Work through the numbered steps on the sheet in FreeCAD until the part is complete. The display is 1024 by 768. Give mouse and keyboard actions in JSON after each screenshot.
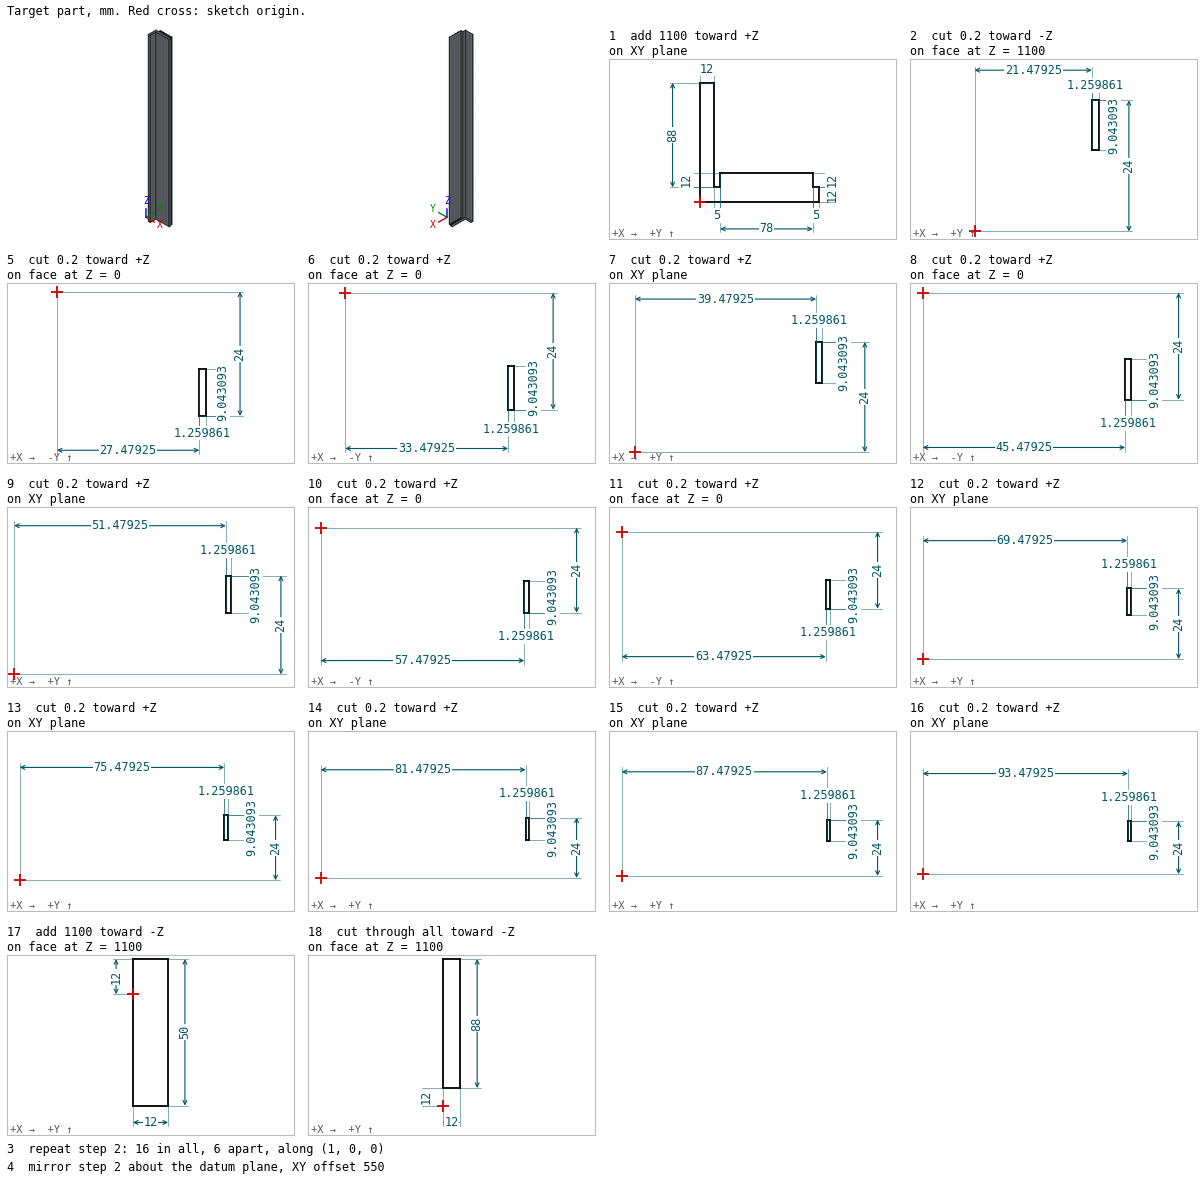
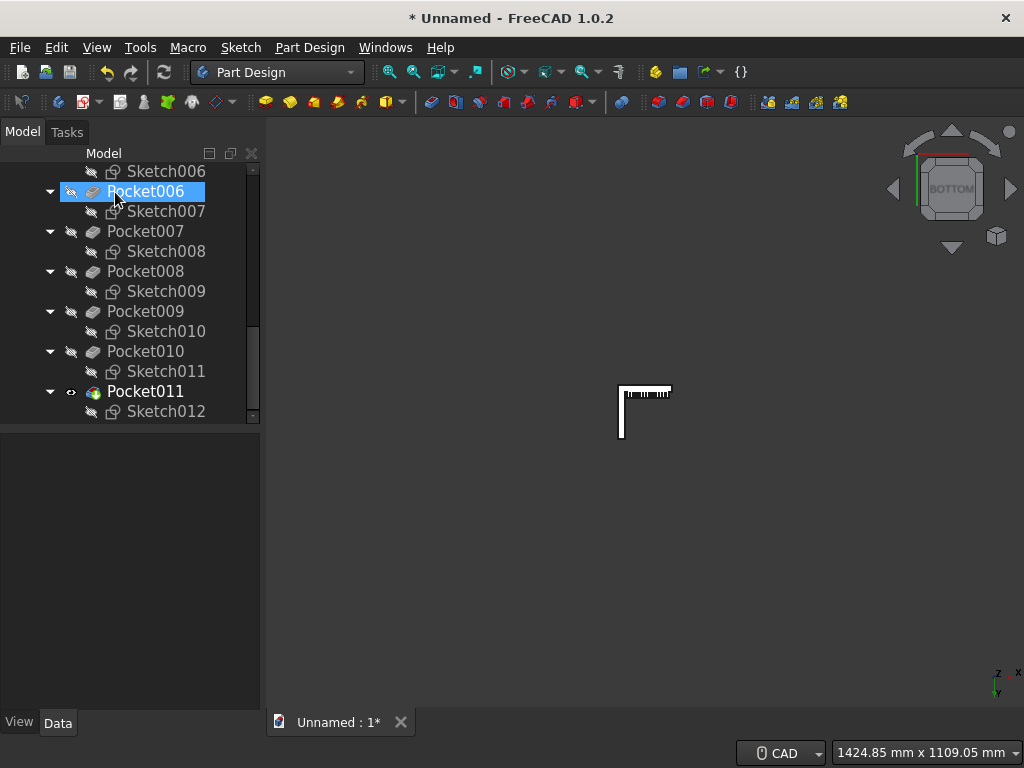
{"action": "left_click", "coordinate": [390, 72]}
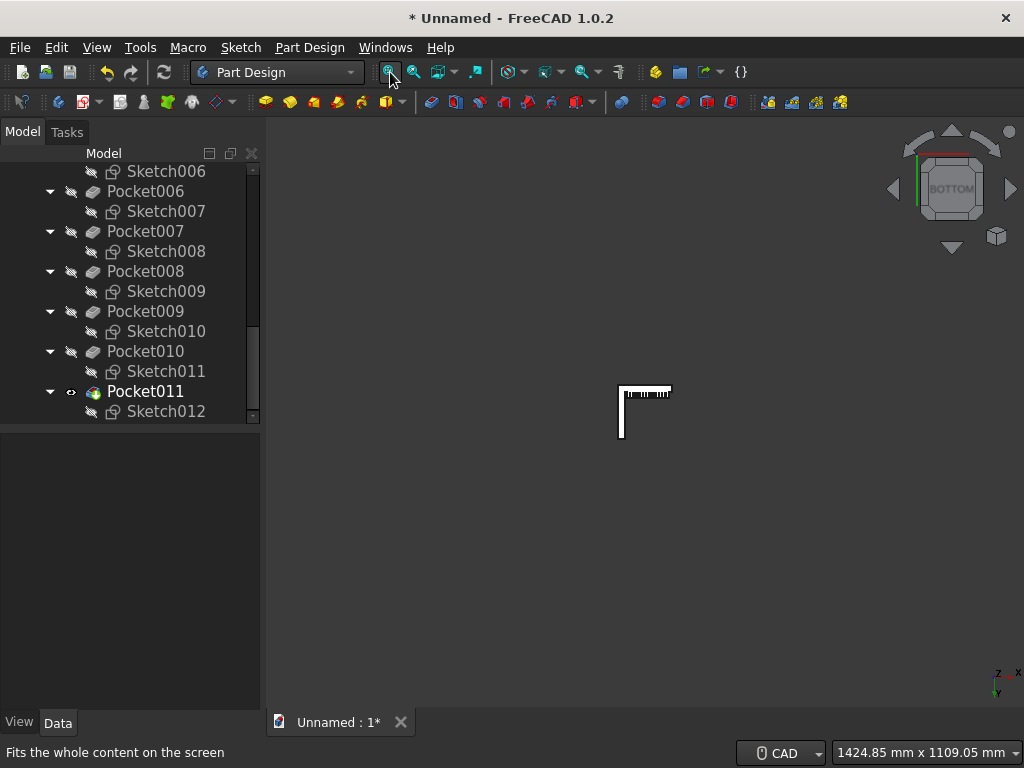
{"action": "left_click", "coordinate": [84, 102]}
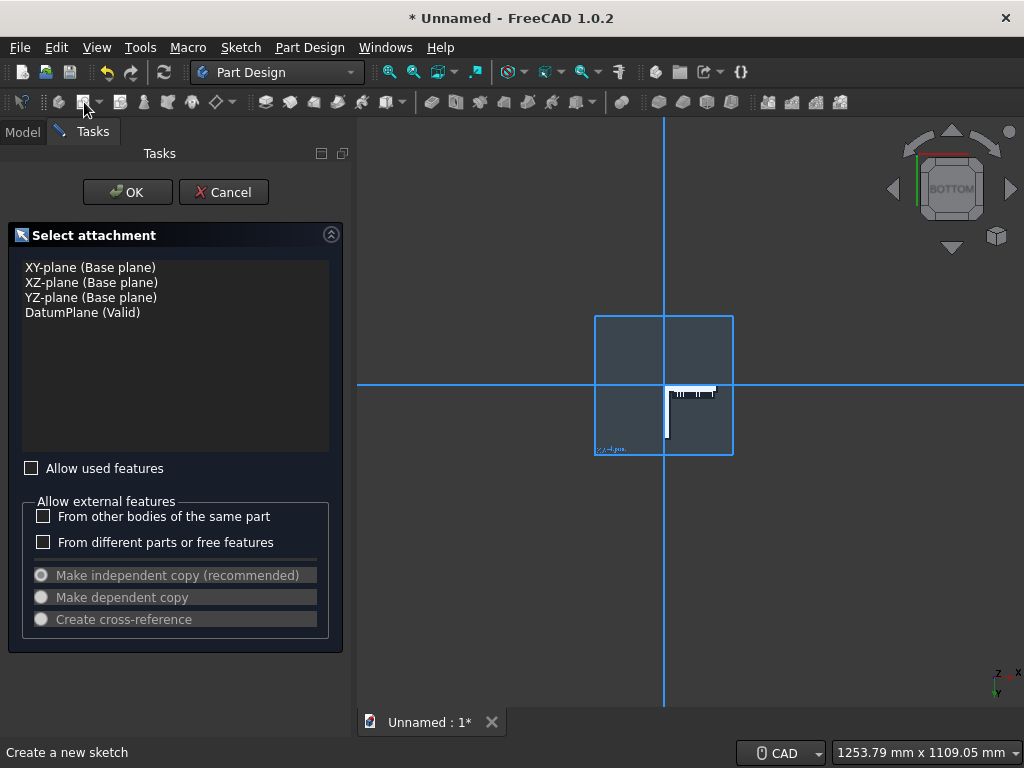
{"action": "left_click", "coordinate": [82, 268]}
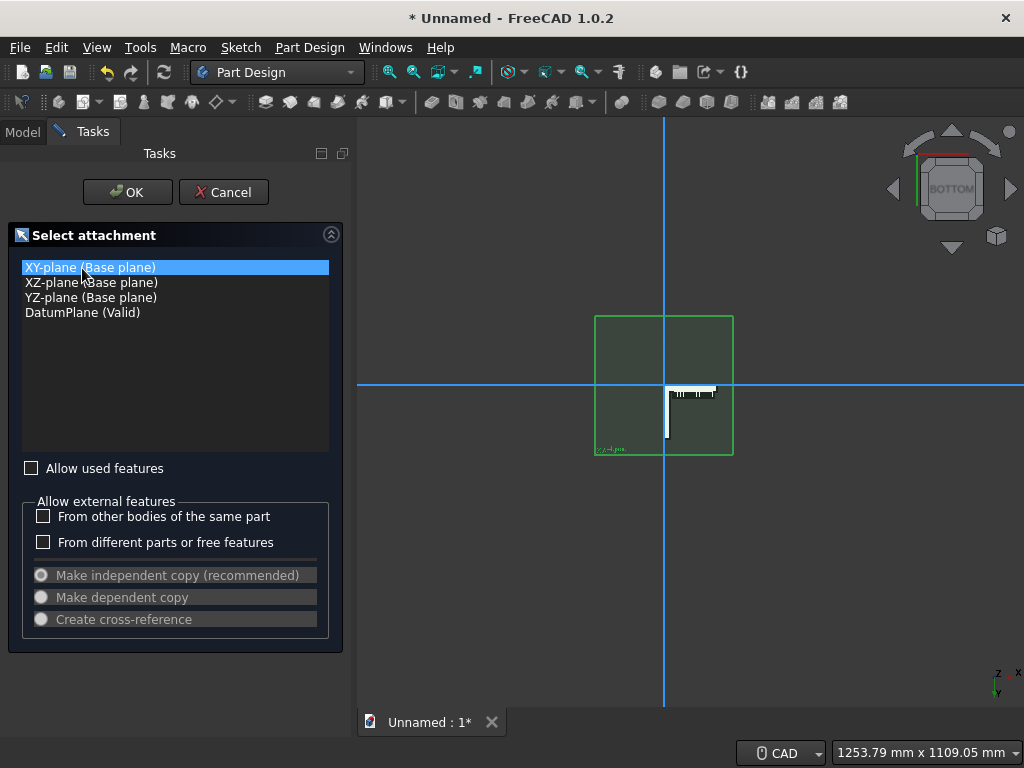
{"action": "left_click", "coordinate": [128, 192]}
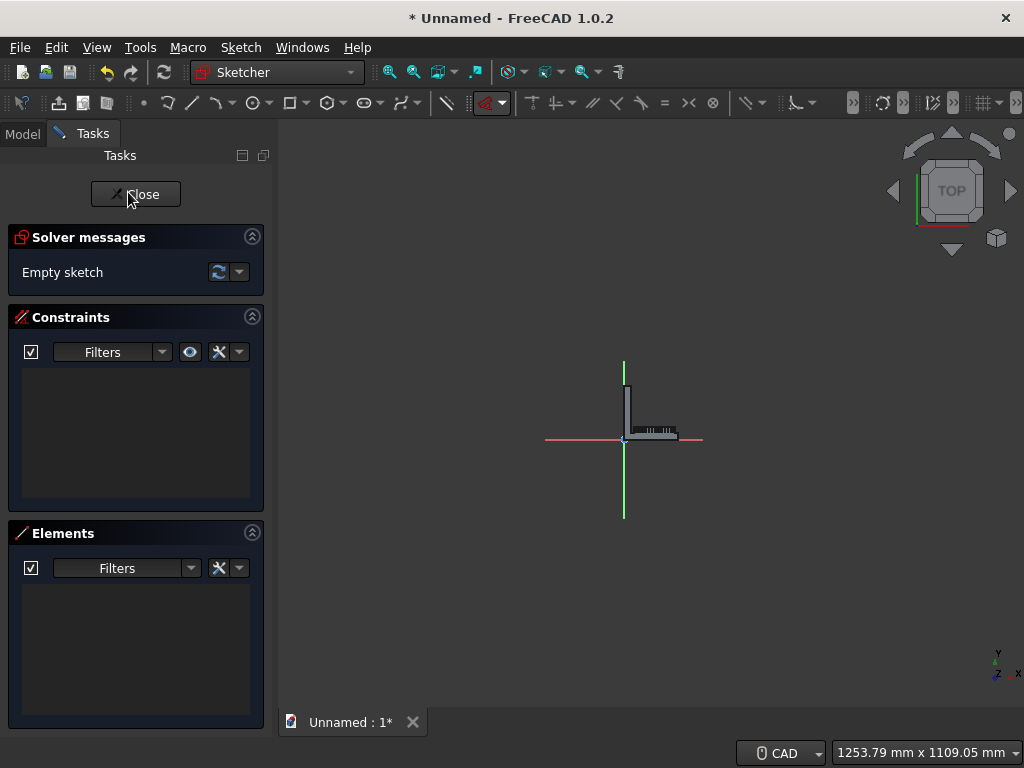
{"action": "left_click", "coordinate": [108, 104]}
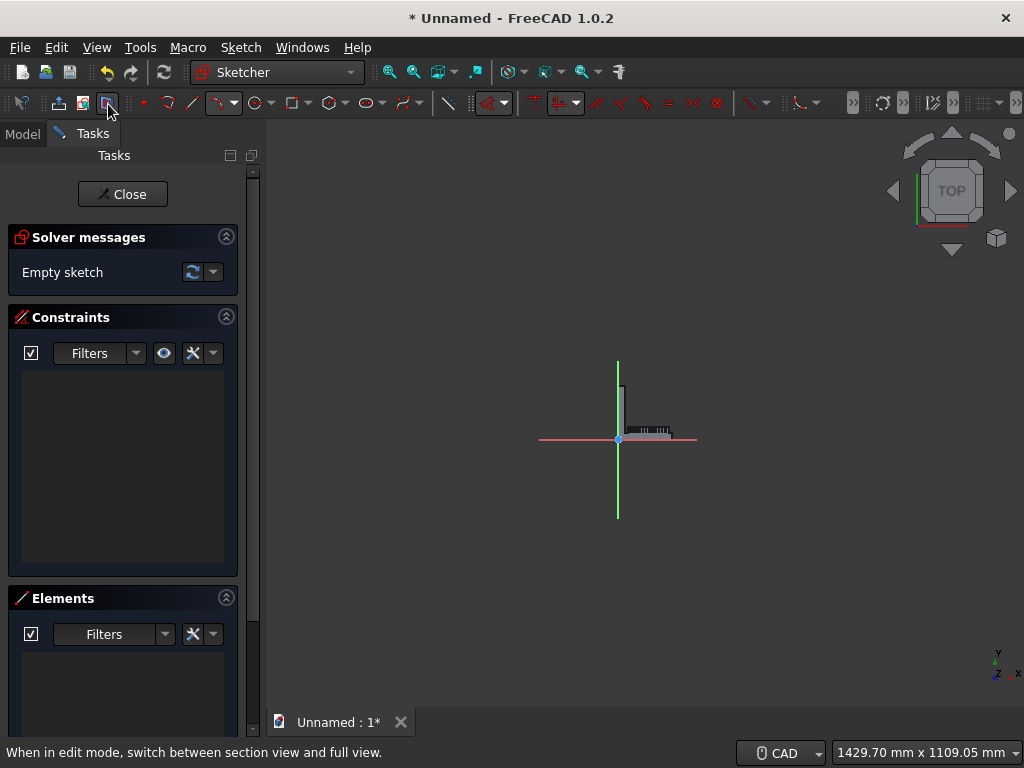
{"action": "scroll", "coordinate": [673, 430], "scroll_direction": "up", "scroll_amount": 15}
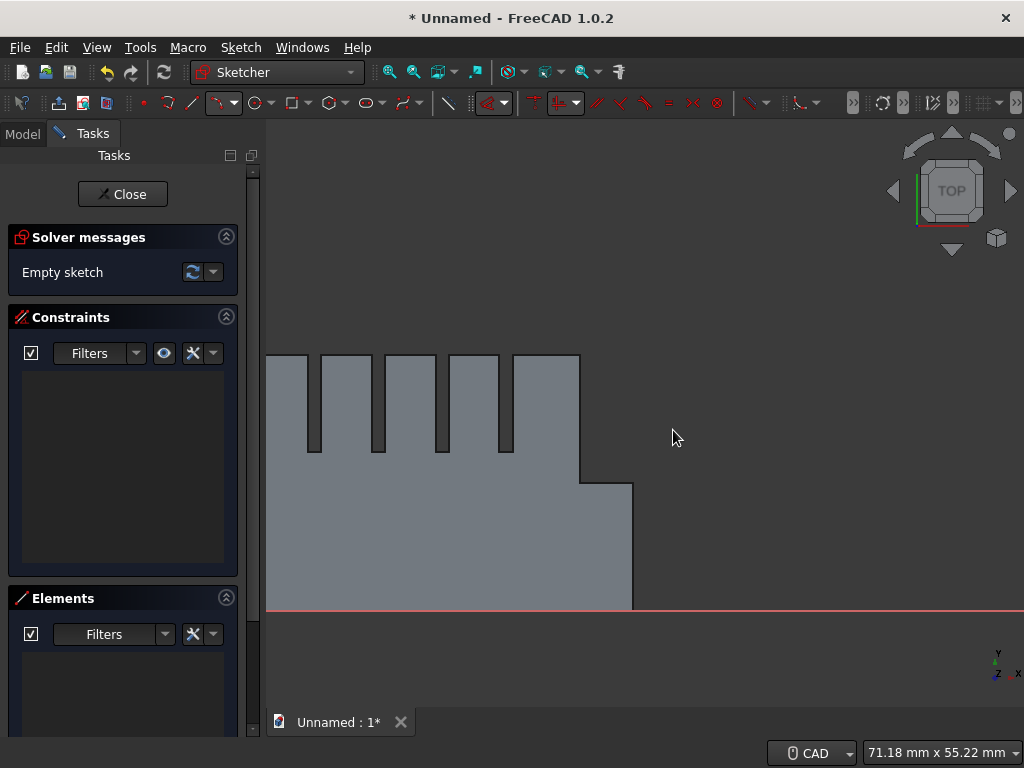
{"action": "scroll", "coordinate": [568, 400], "scroll_direction": "up", "scroll_amount": 7}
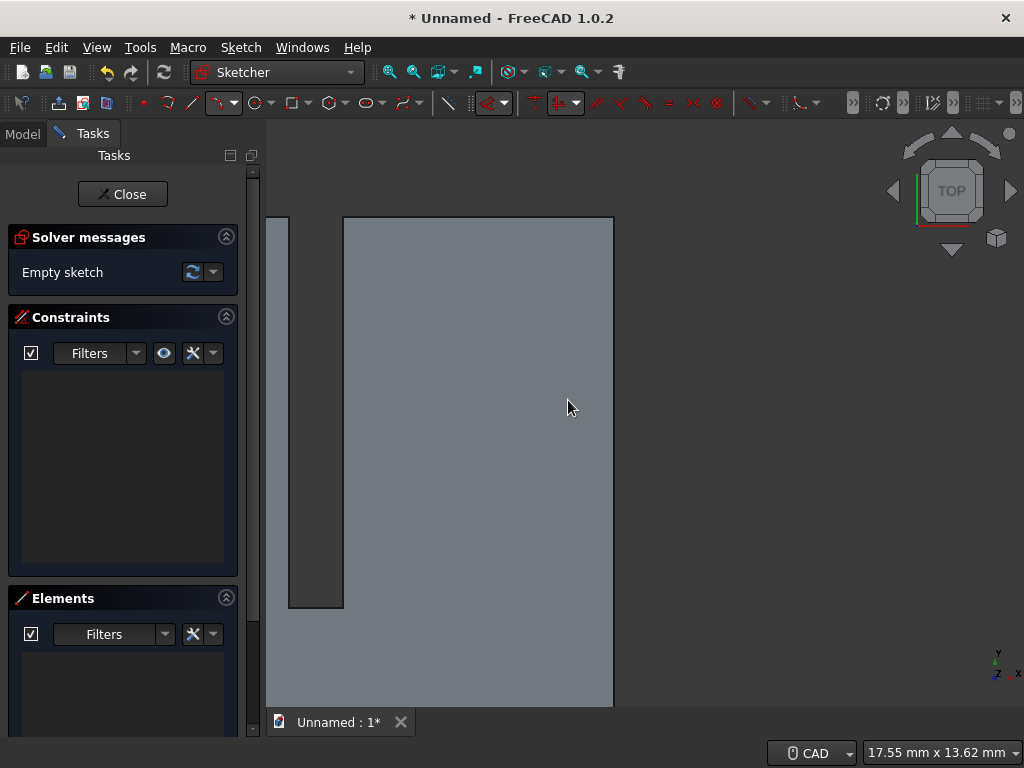
{"action": "left_click", "coordinate": [292, 104]}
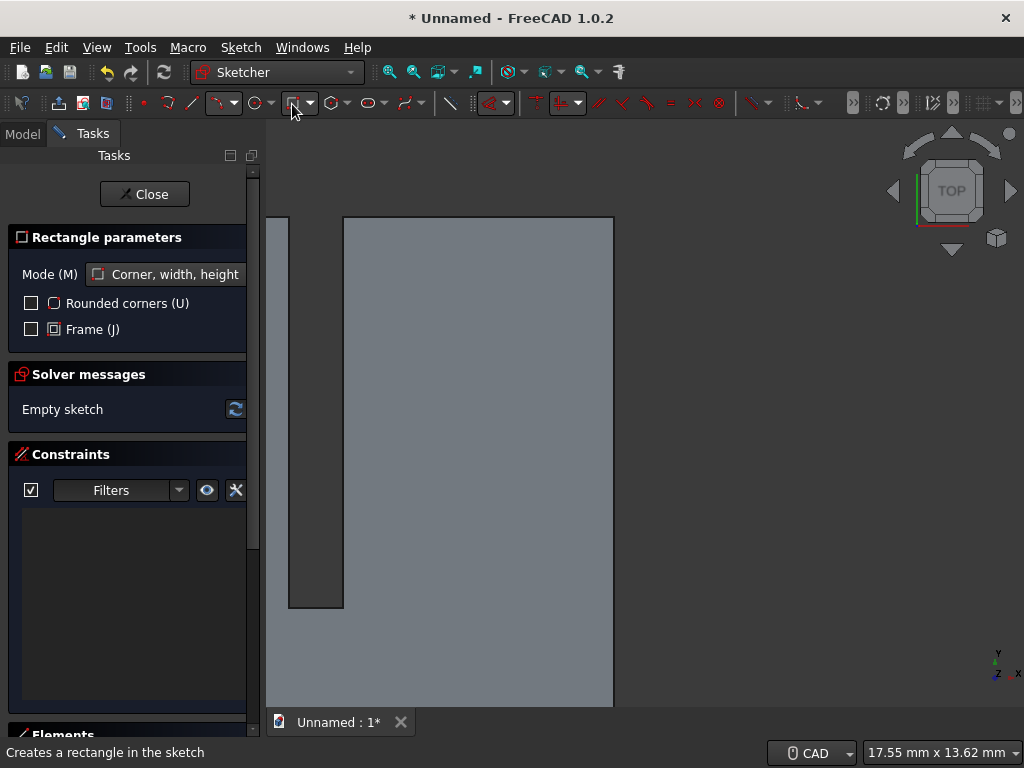
{"action": "left_click", "coordinate": [548, 217]}
{"action": "mouse_move", "coordinate": [602, 608]}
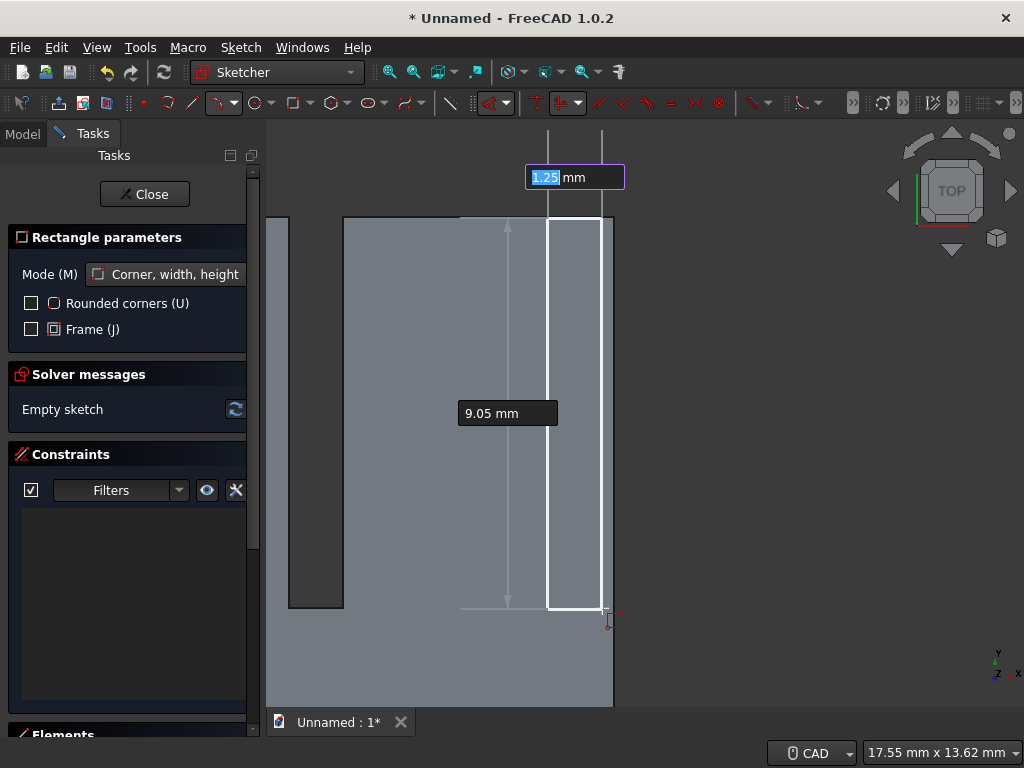
{"action": "type", "text": "1.259861"}
{"action": "key", "text": "Tab"}
{"action": "type", "text": "9.043093"}
{"action": "key", "text": "Return"}
{"action": "key", "text": "Escape"}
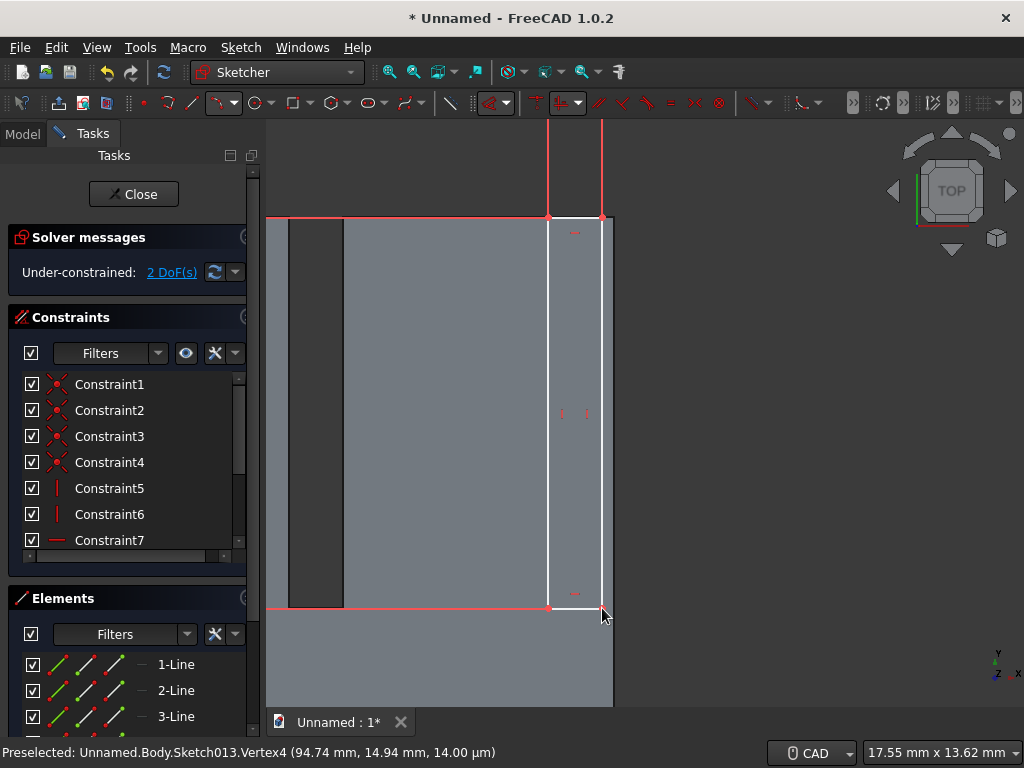
{"action": "left_click", "coordinate": [548, 218]}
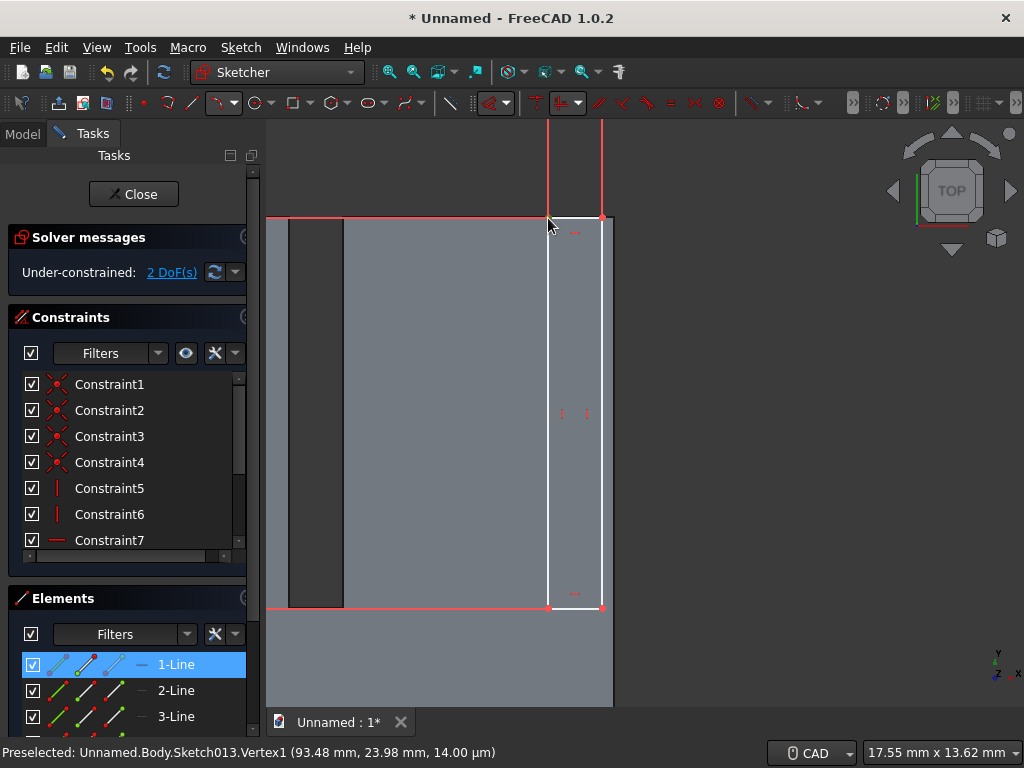
{"action": "key", "text": "i"}